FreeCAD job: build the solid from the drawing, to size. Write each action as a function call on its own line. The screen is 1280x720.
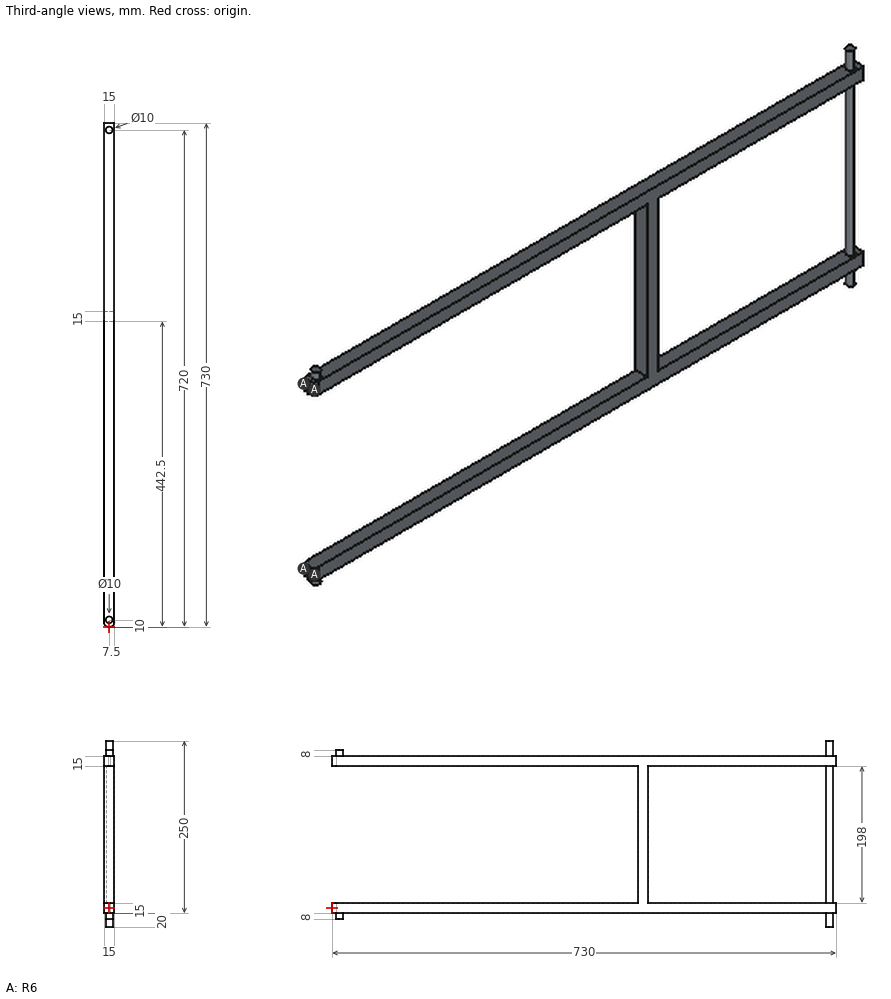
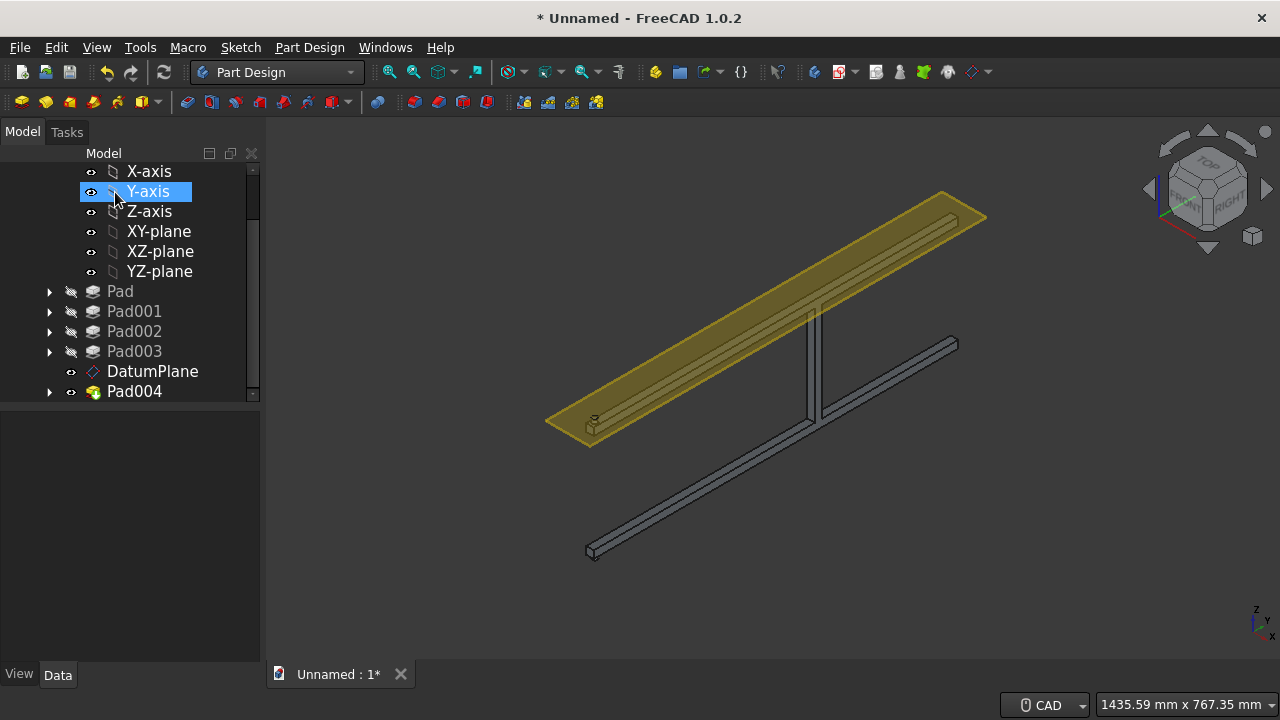
click(116, 372)
key(space)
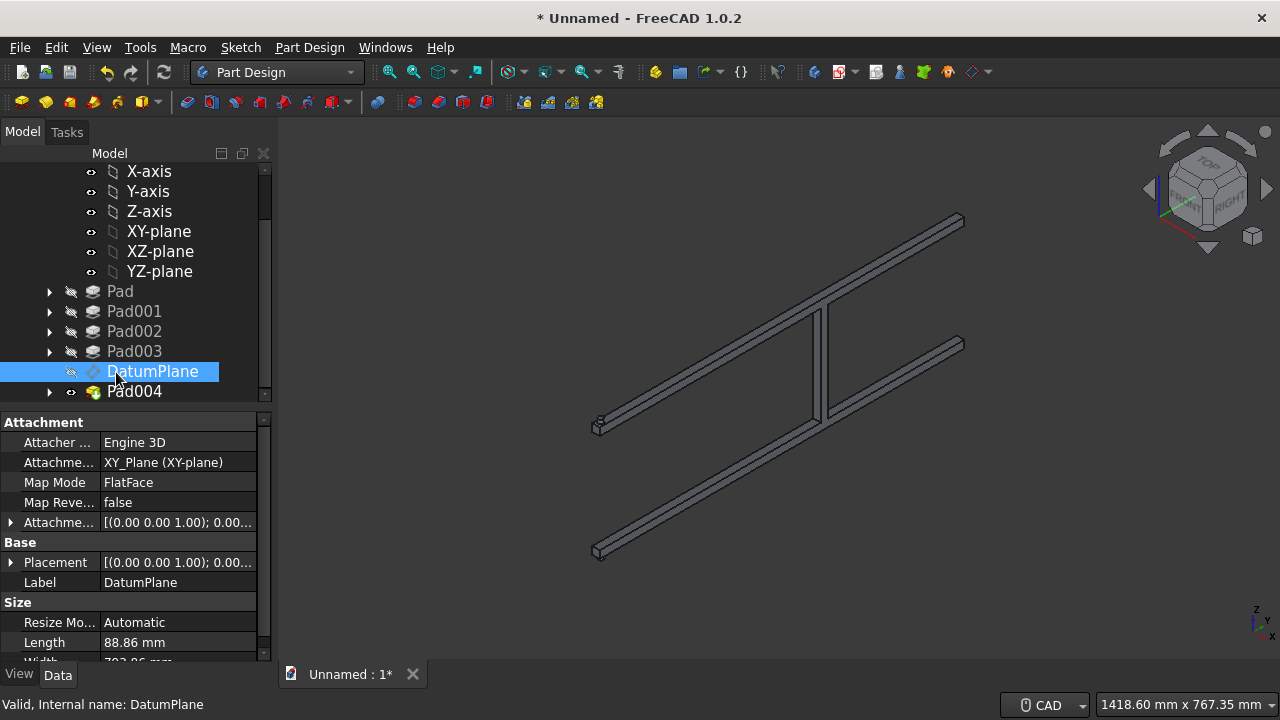
click(600, 433)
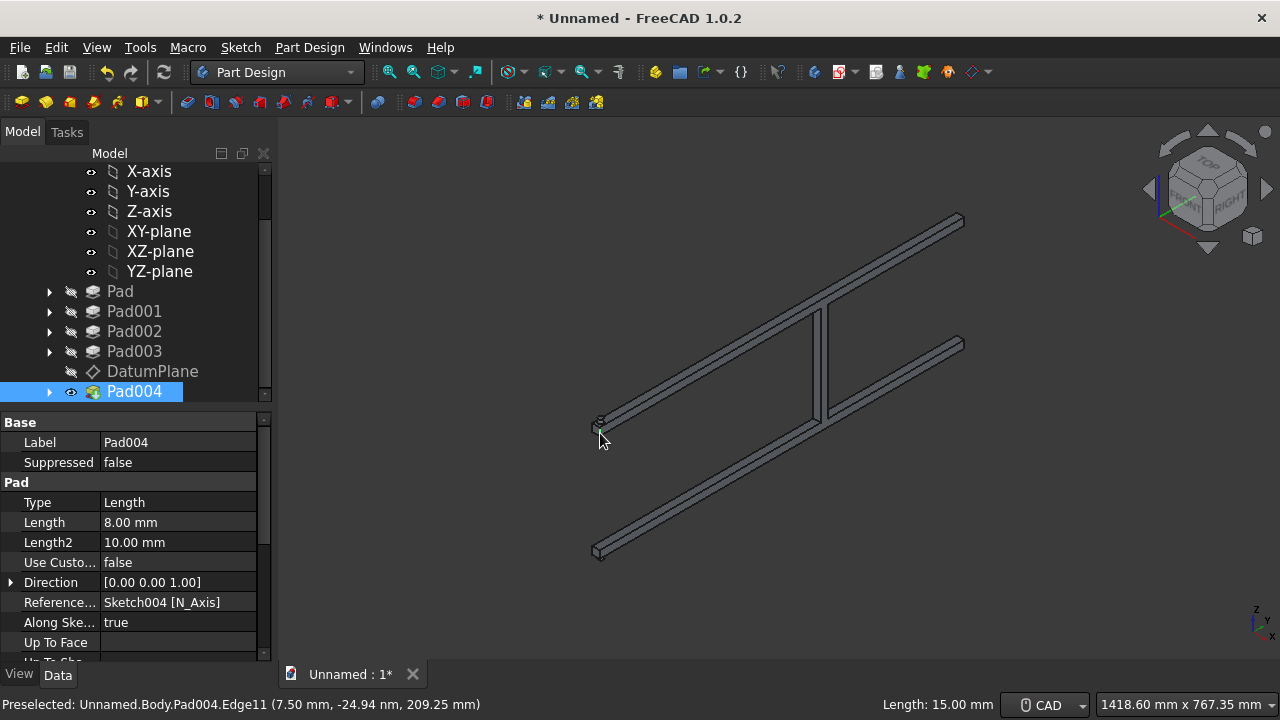
click(600, 556, ctrl)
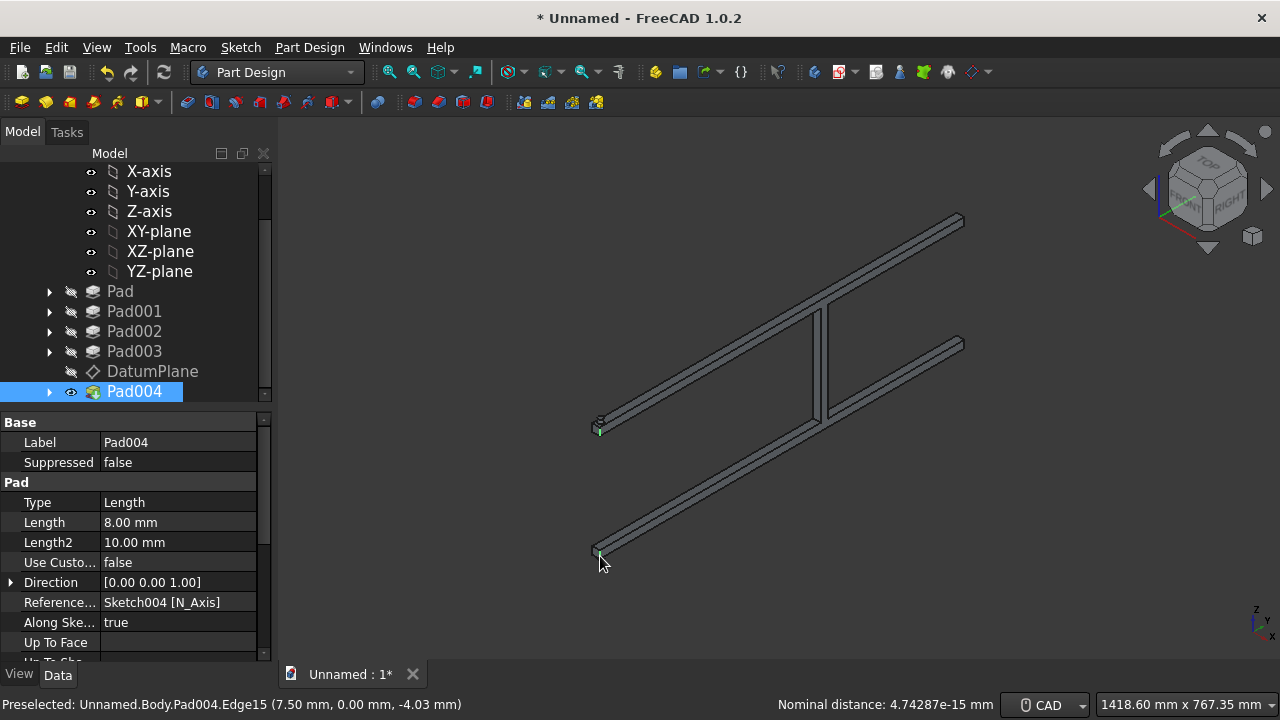
scroll(592, 427, up, 7)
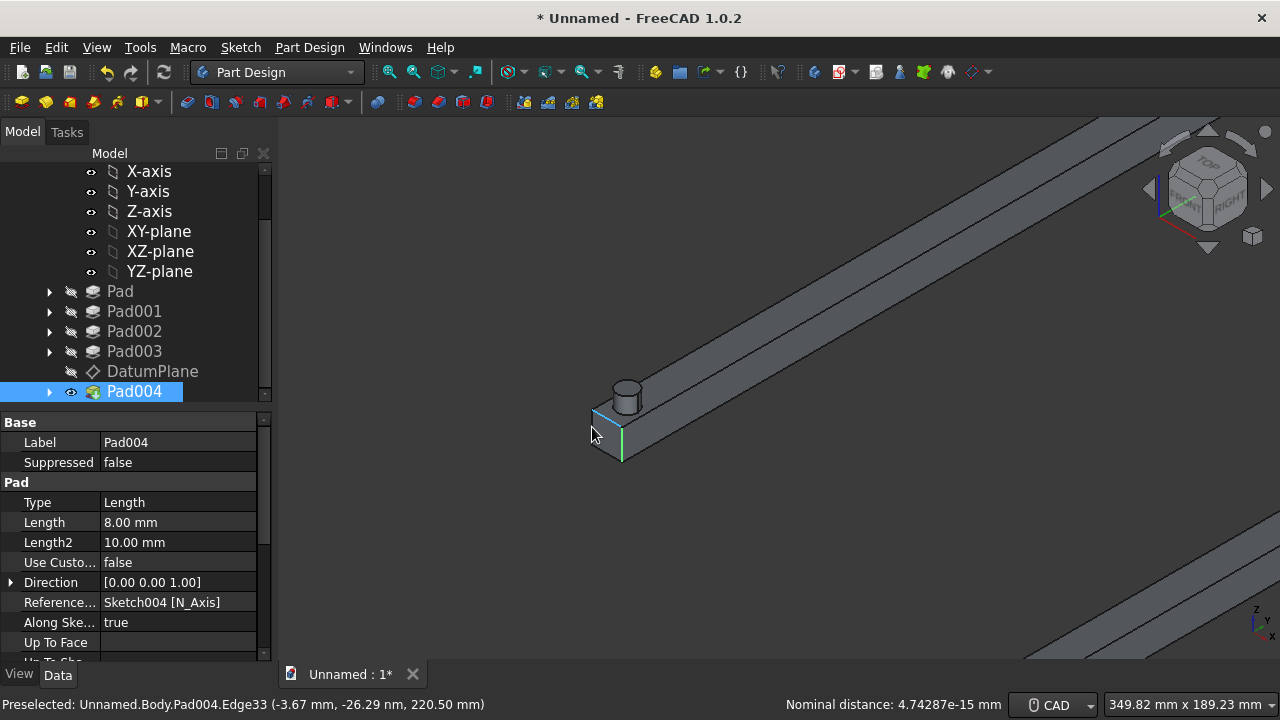
click(390, 72)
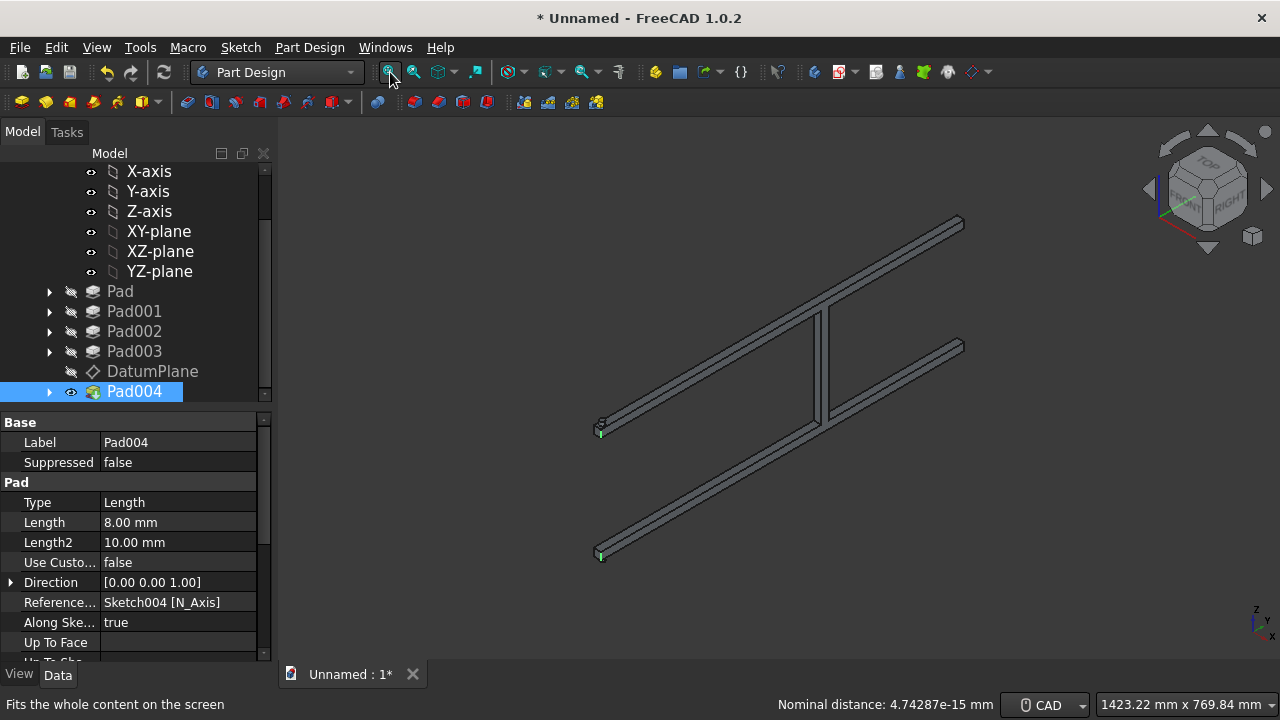
key(2)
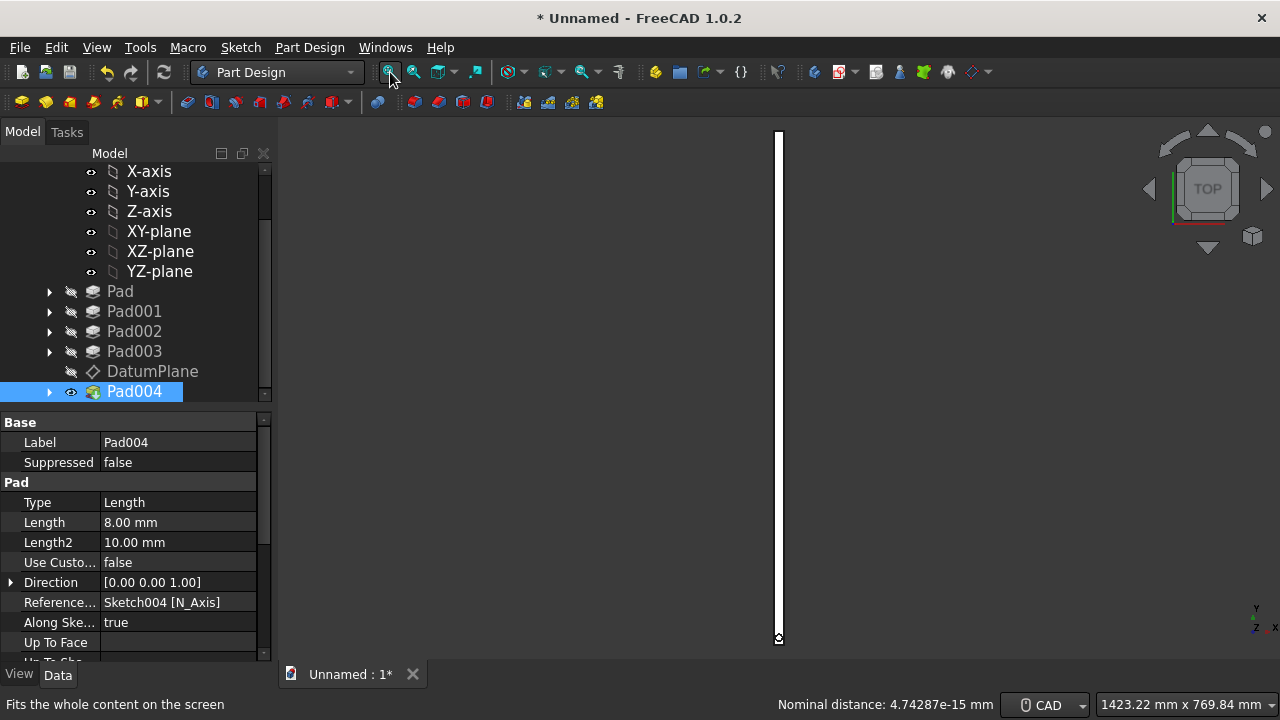
key(0)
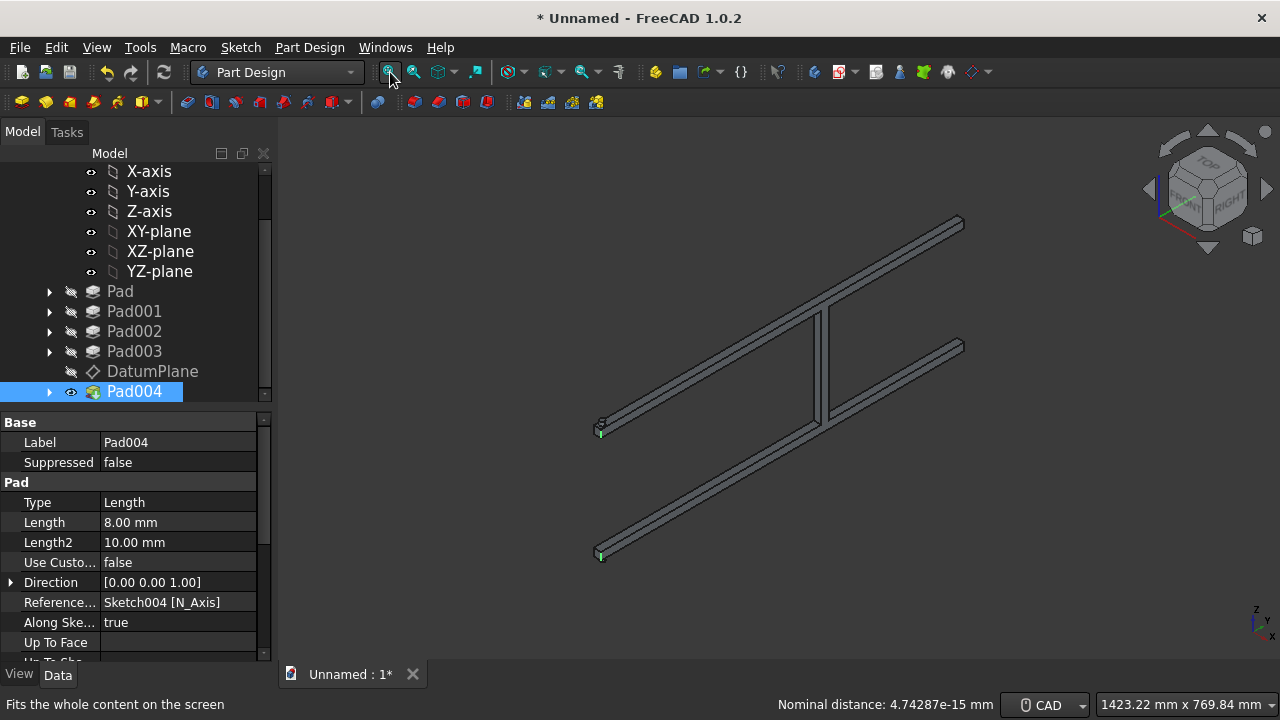
scroll(594, 429, up, 7)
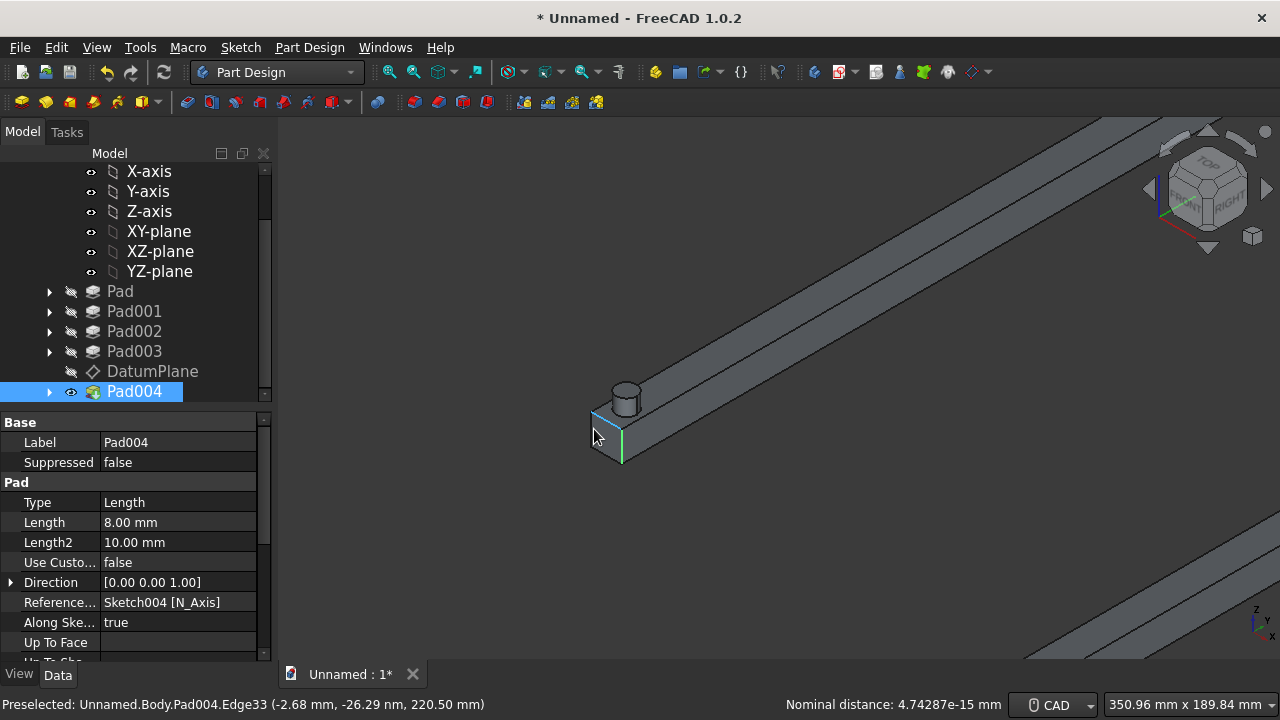
key(v)
key(f)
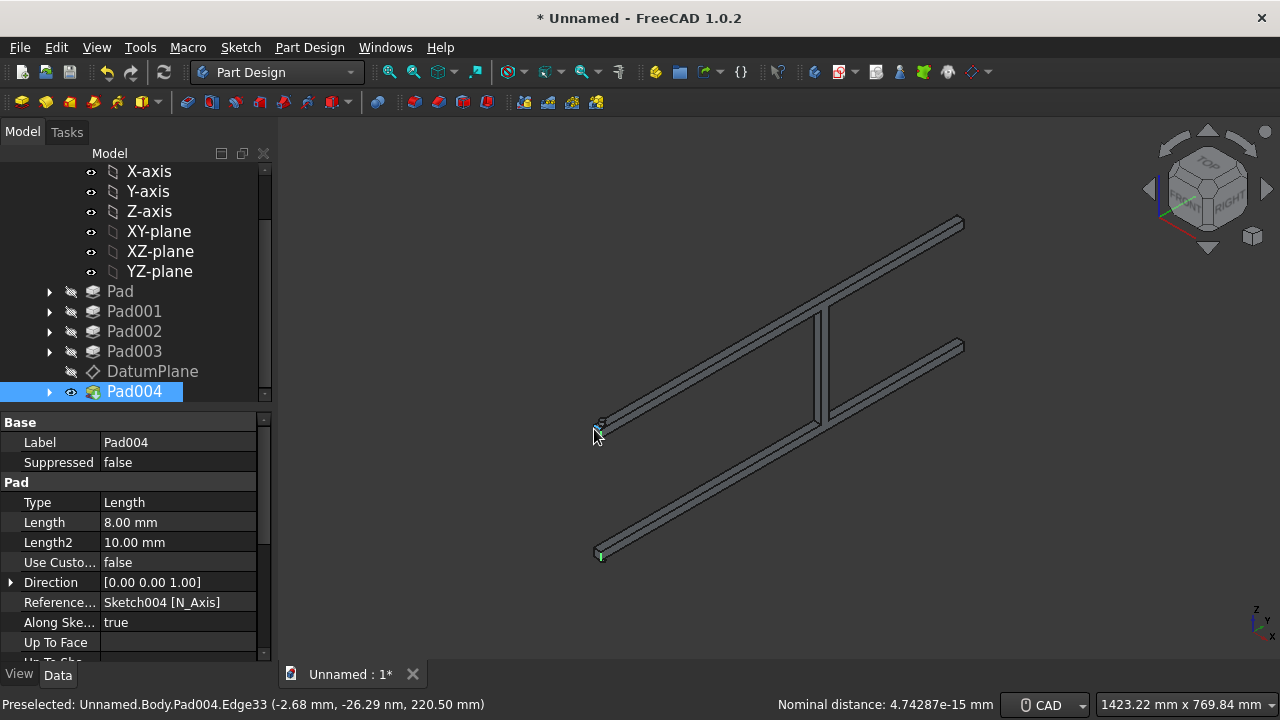
key(1)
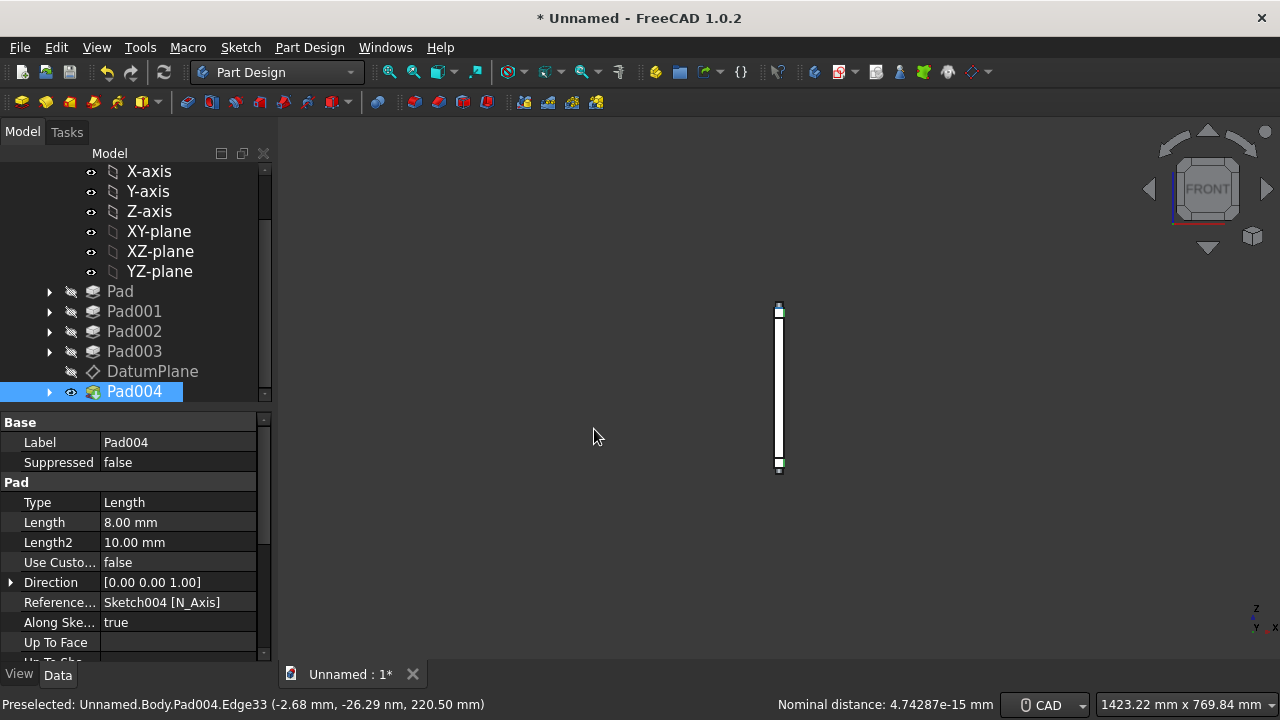
click(390, 72)